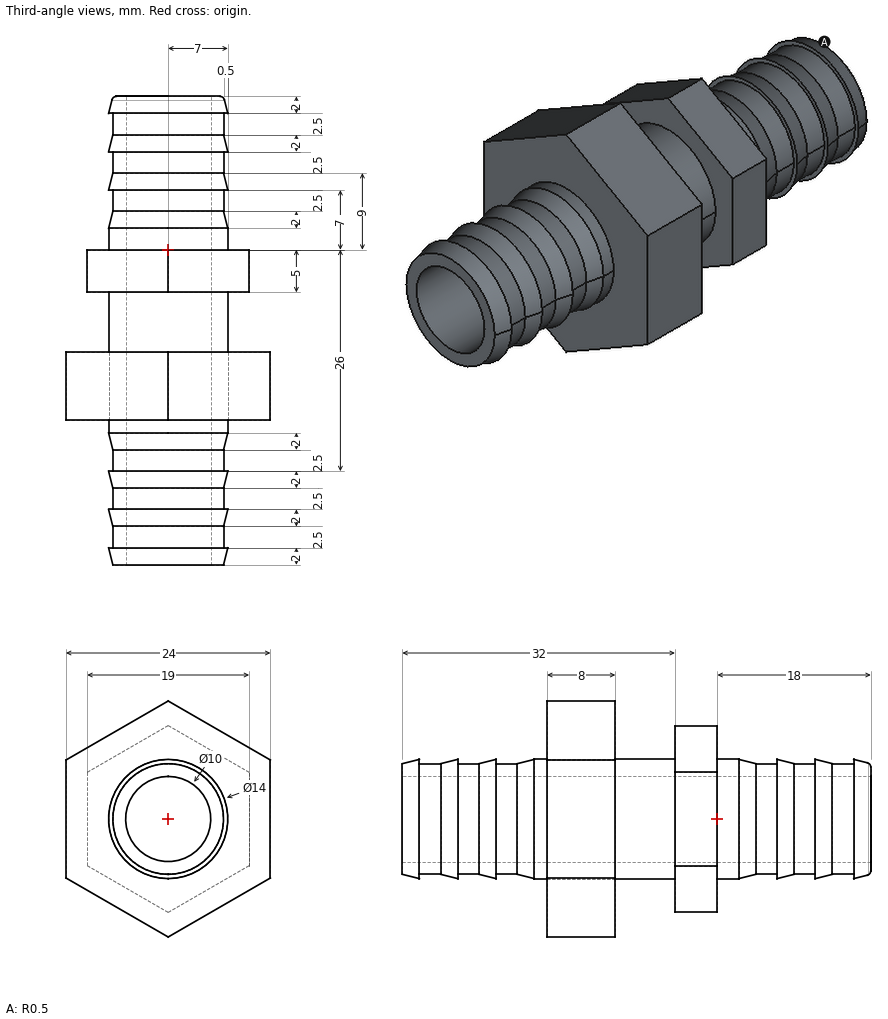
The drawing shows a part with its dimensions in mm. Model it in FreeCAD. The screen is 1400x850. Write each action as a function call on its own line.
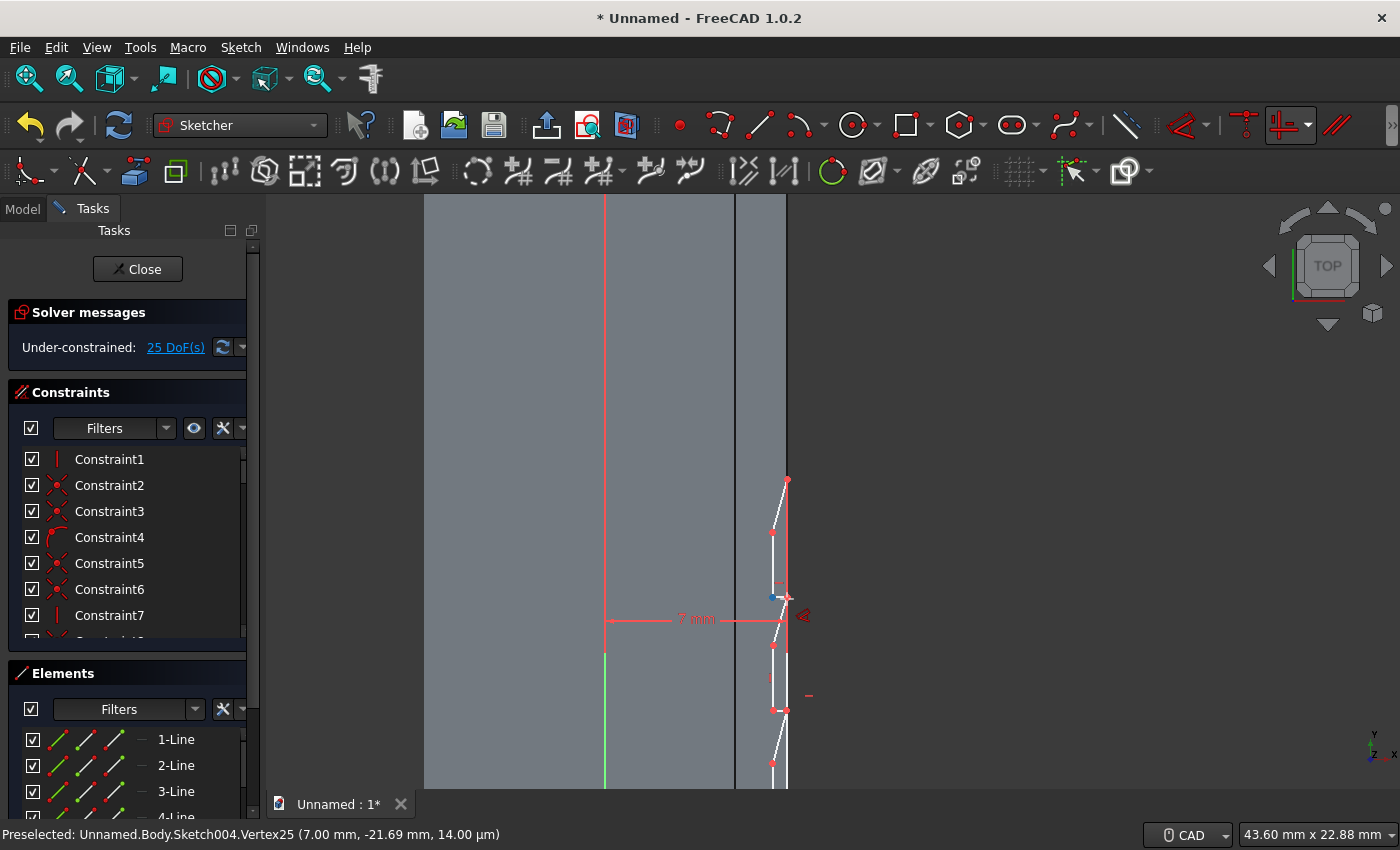
click(787, 597)
click(696, 655)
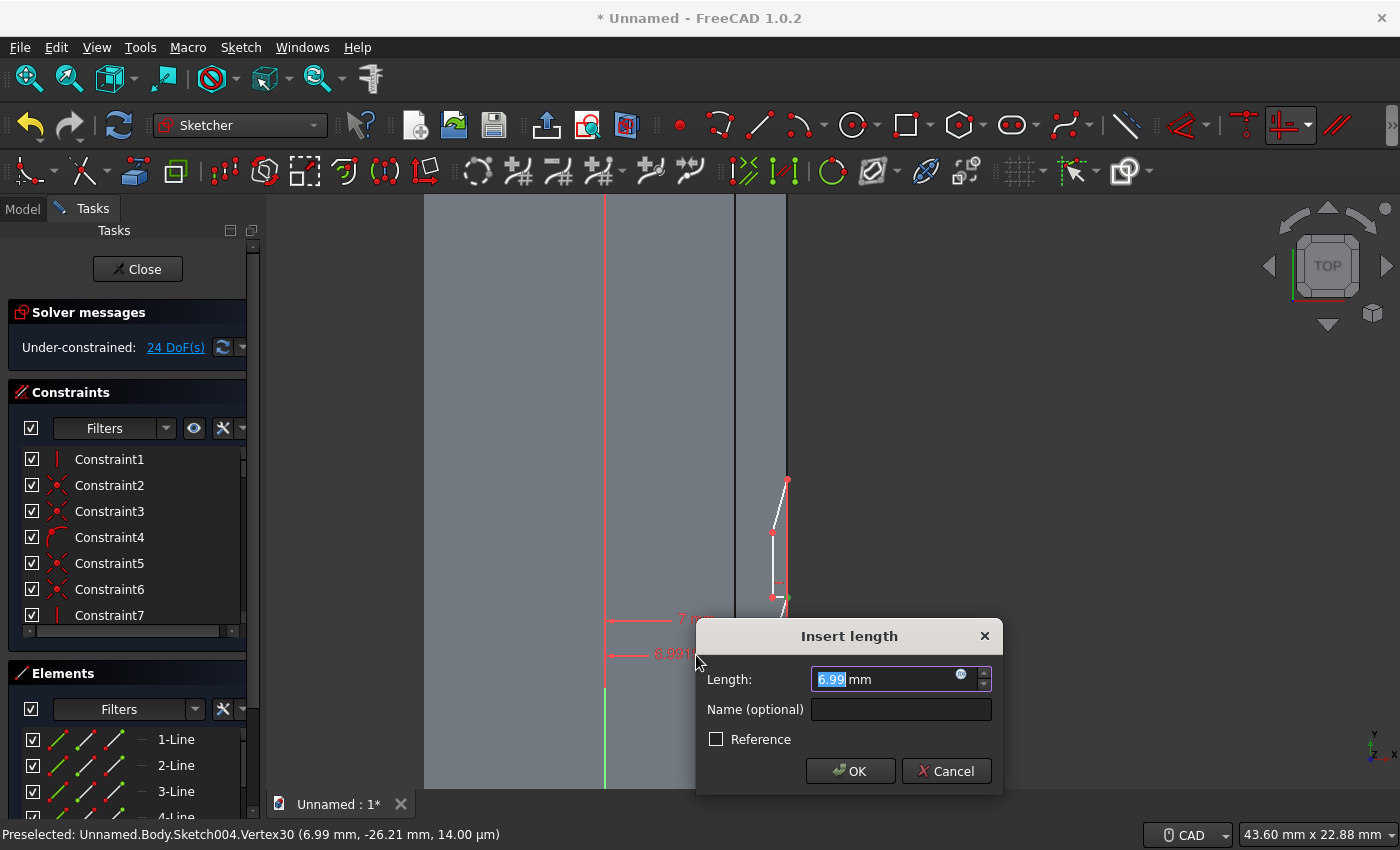
text(7)
key(Return)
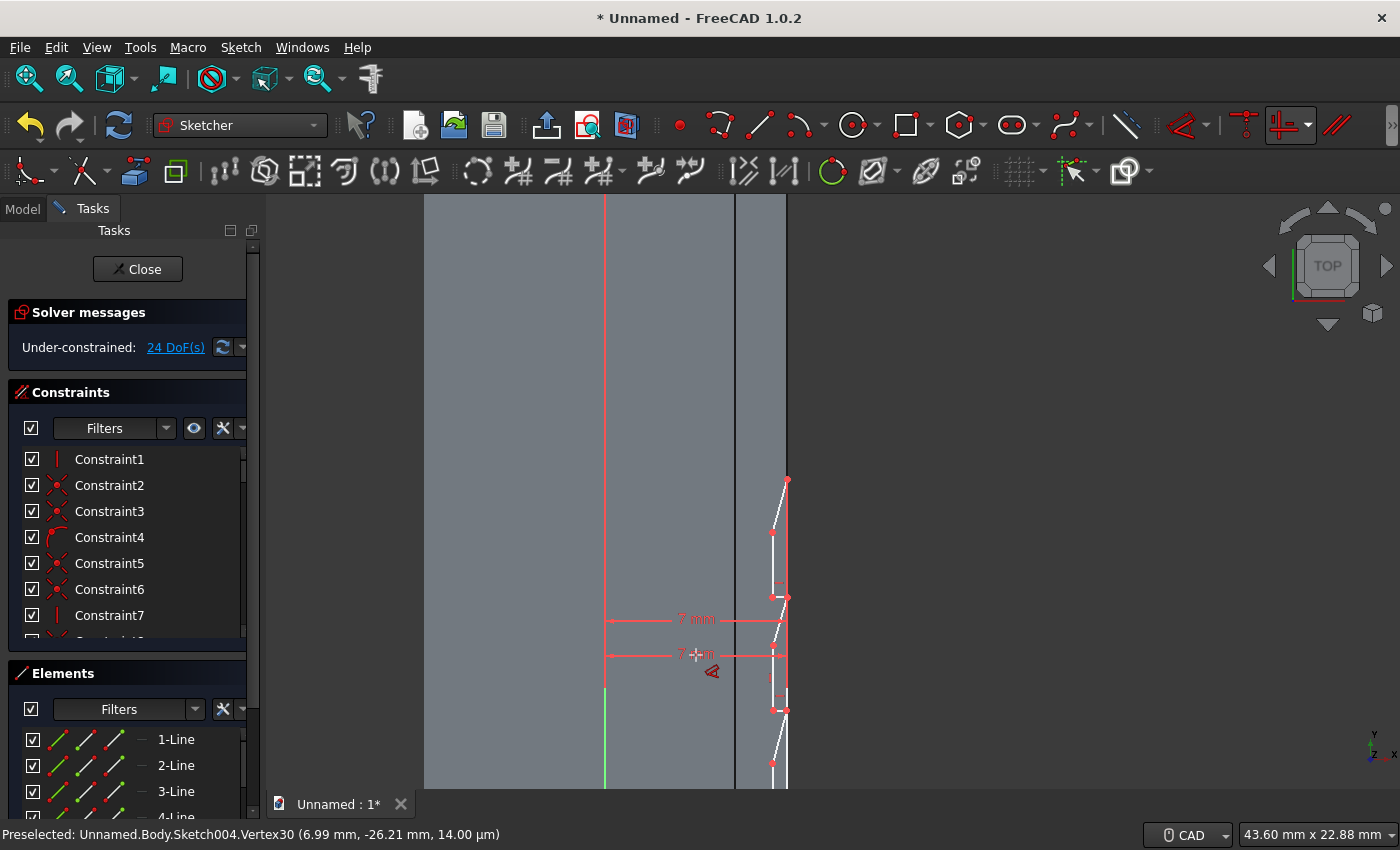
click(787, 711)
click(696, 745)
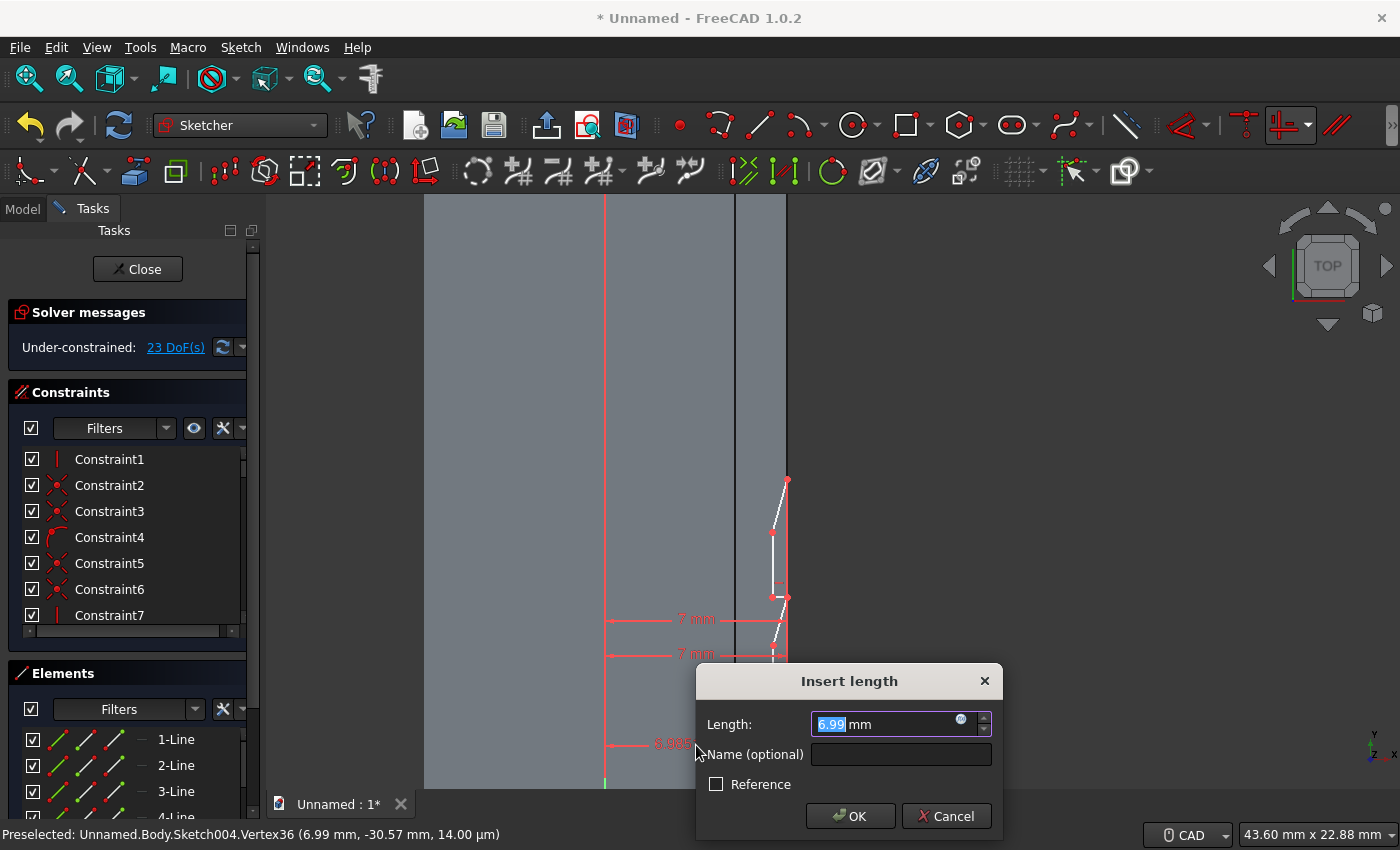
text(7)
key(Return)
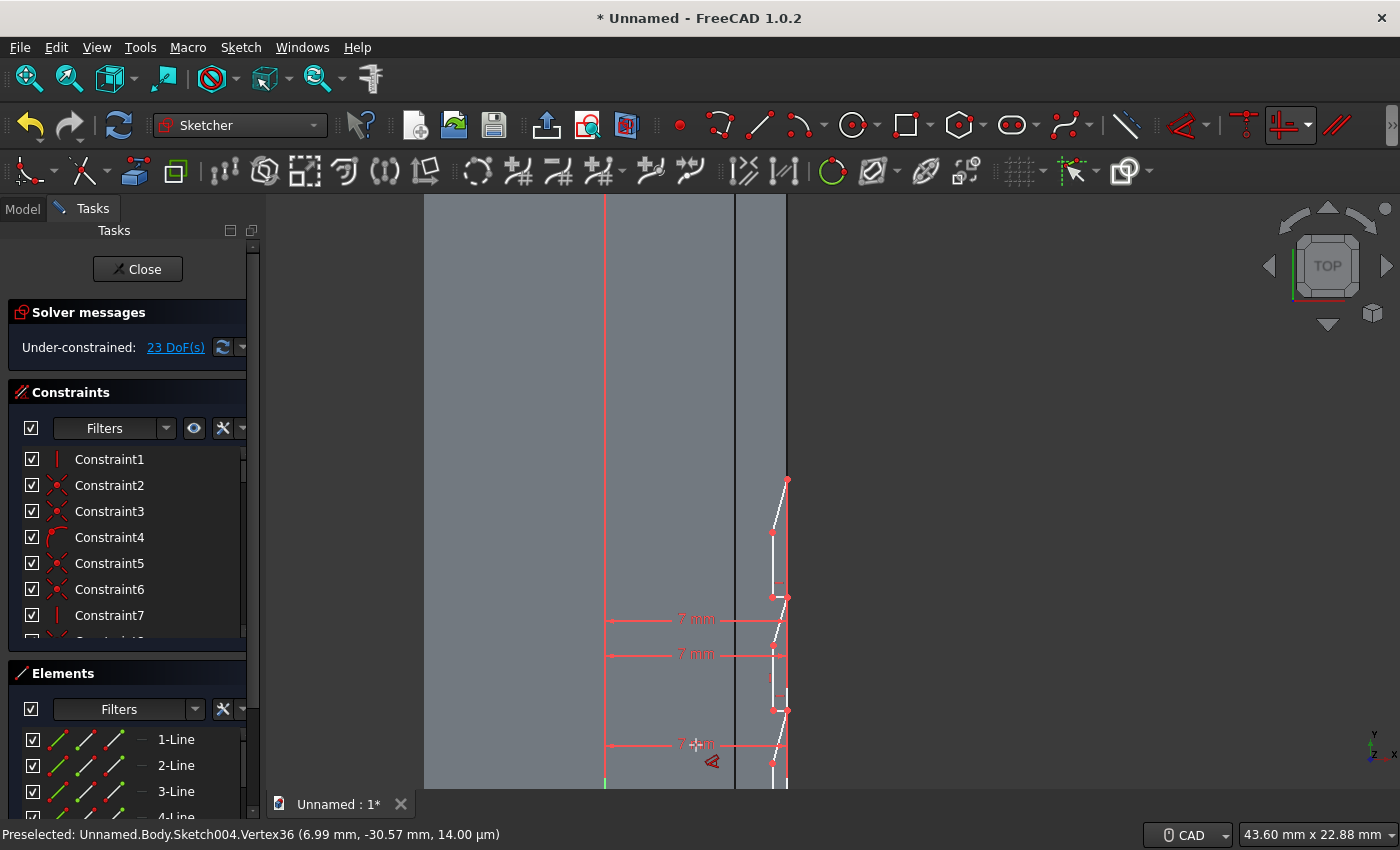
scroll(787, 599, down, 7)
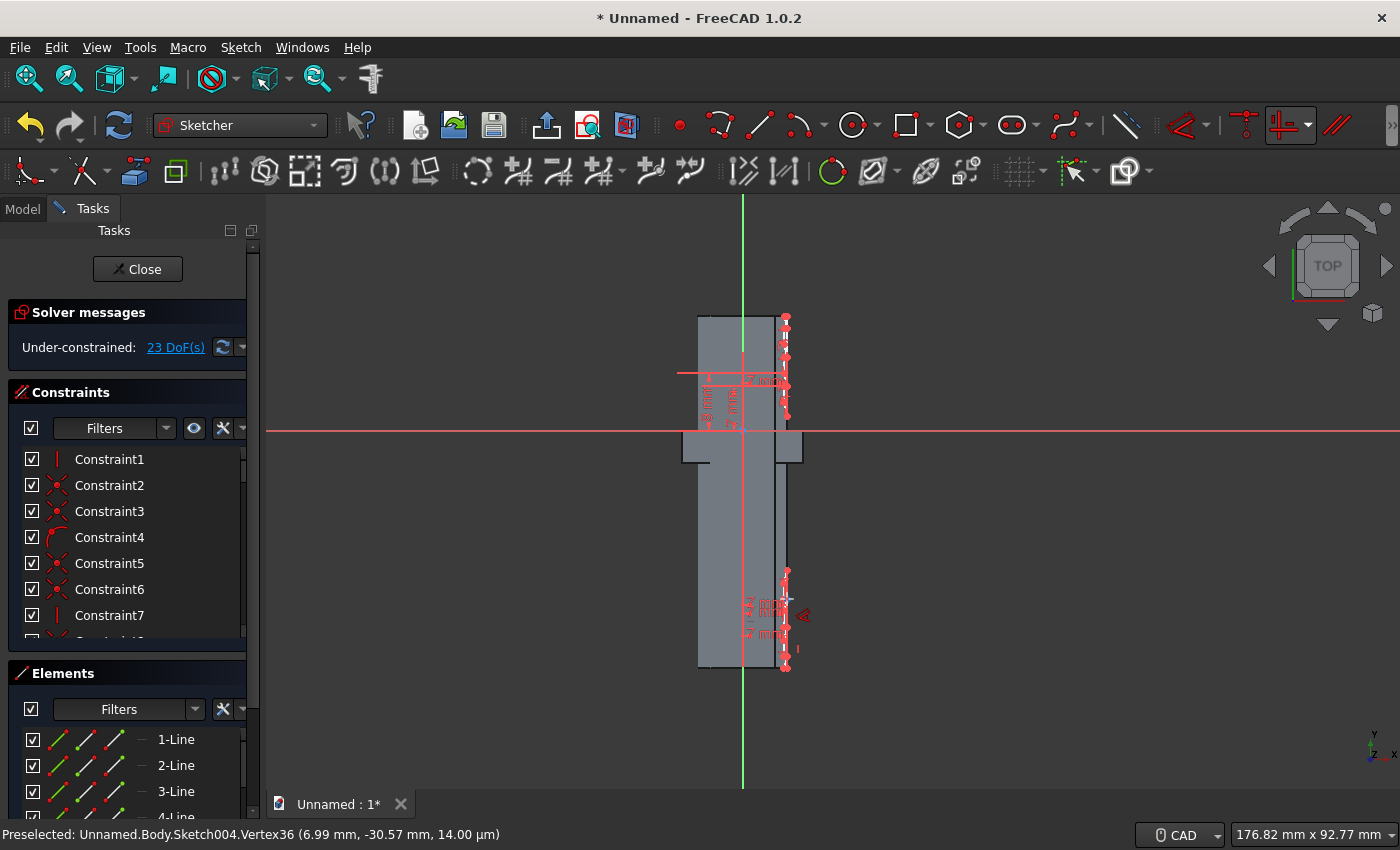
scroll(787, 656, up, 7)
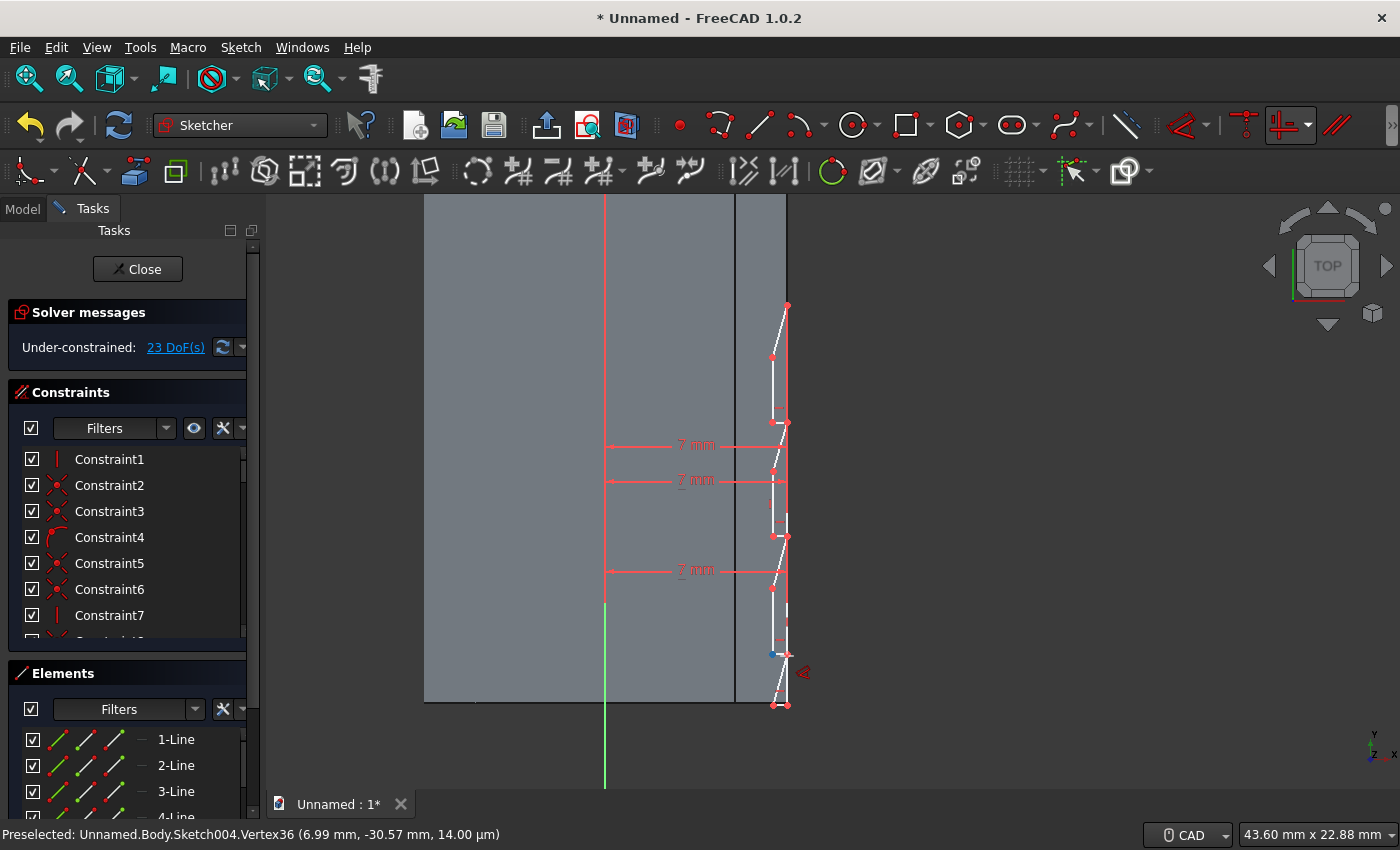
click(787, 654)
click(696, 688)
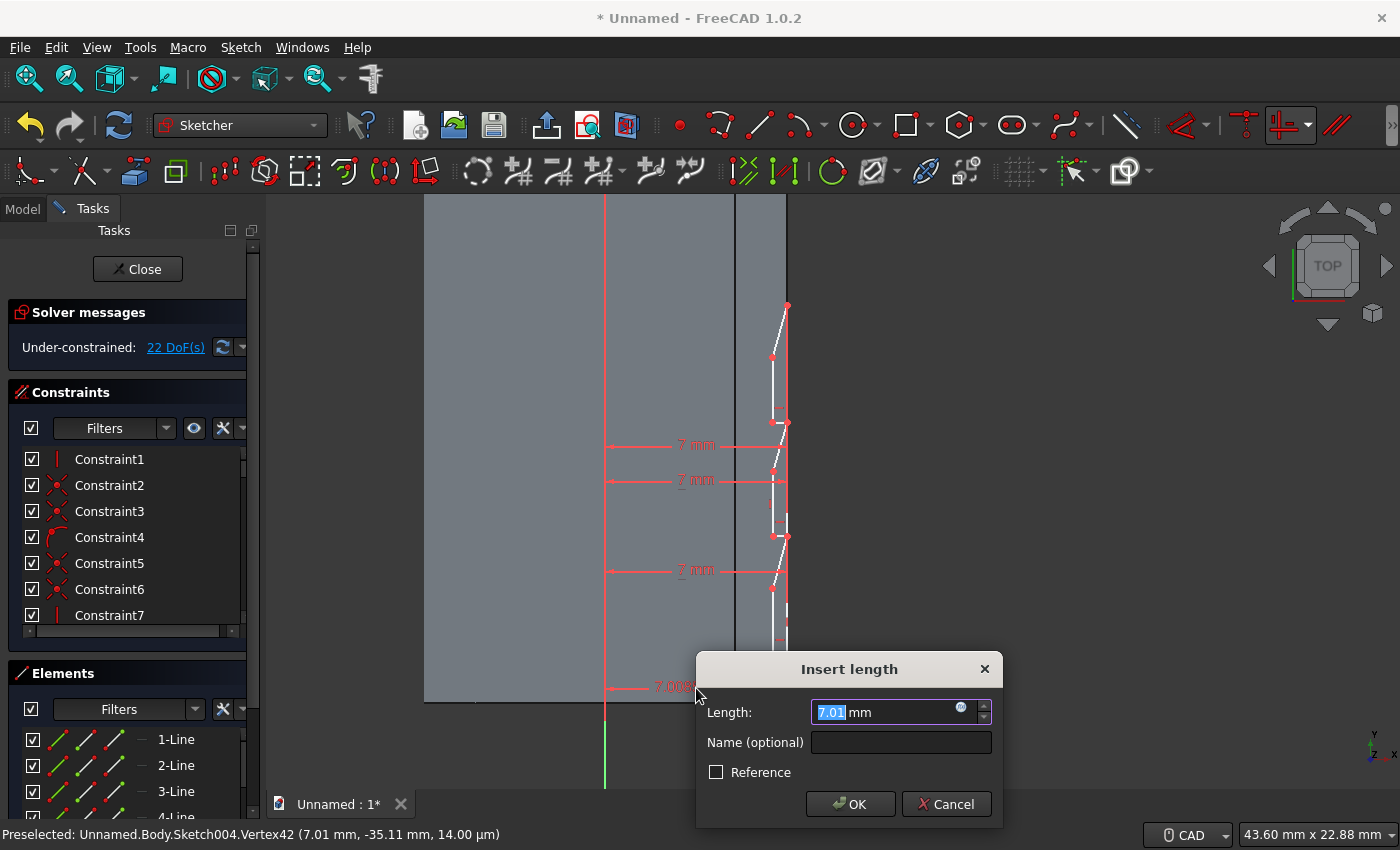
text(7)
key(Return)